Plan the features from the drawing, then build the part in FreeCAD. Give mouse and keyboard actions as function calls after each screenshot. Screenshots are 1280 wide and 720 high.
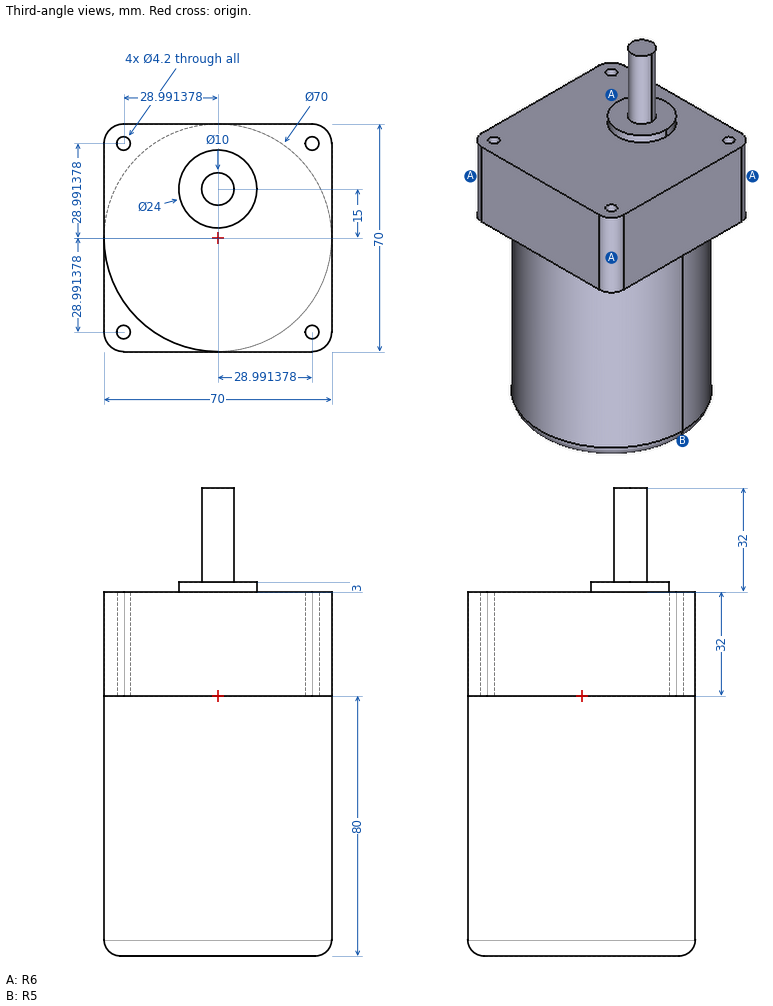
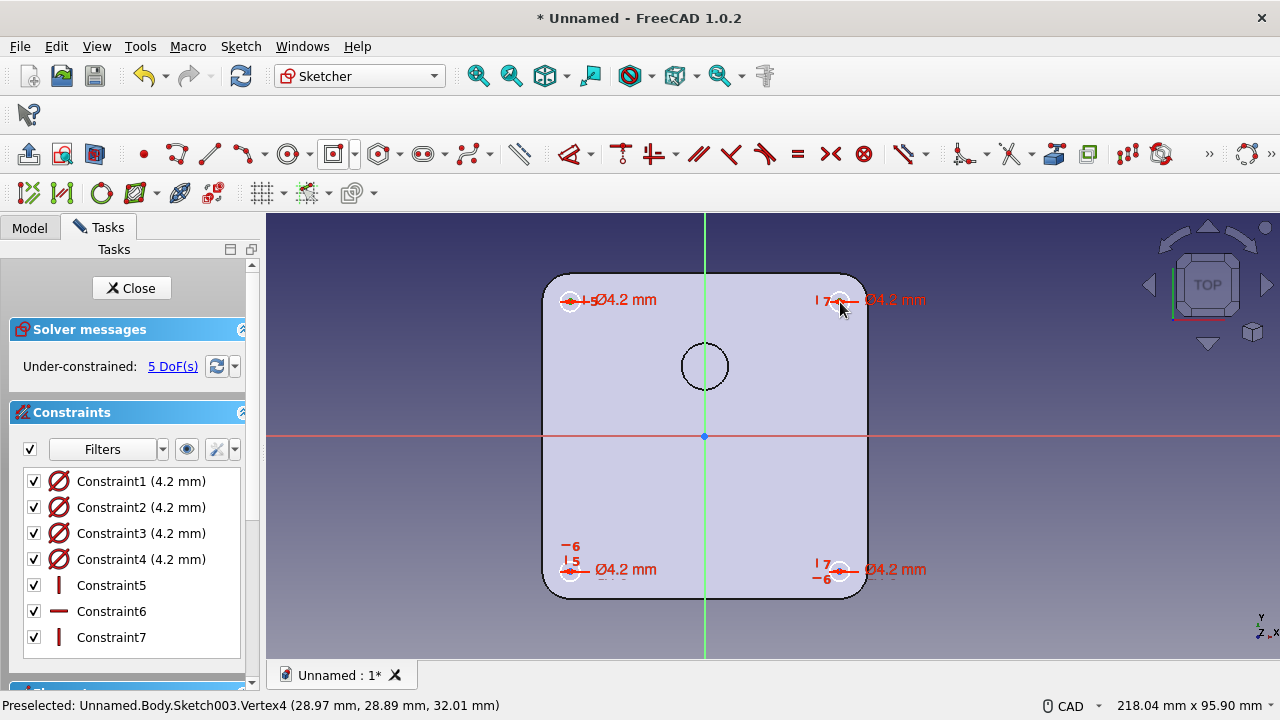
click(676, 154)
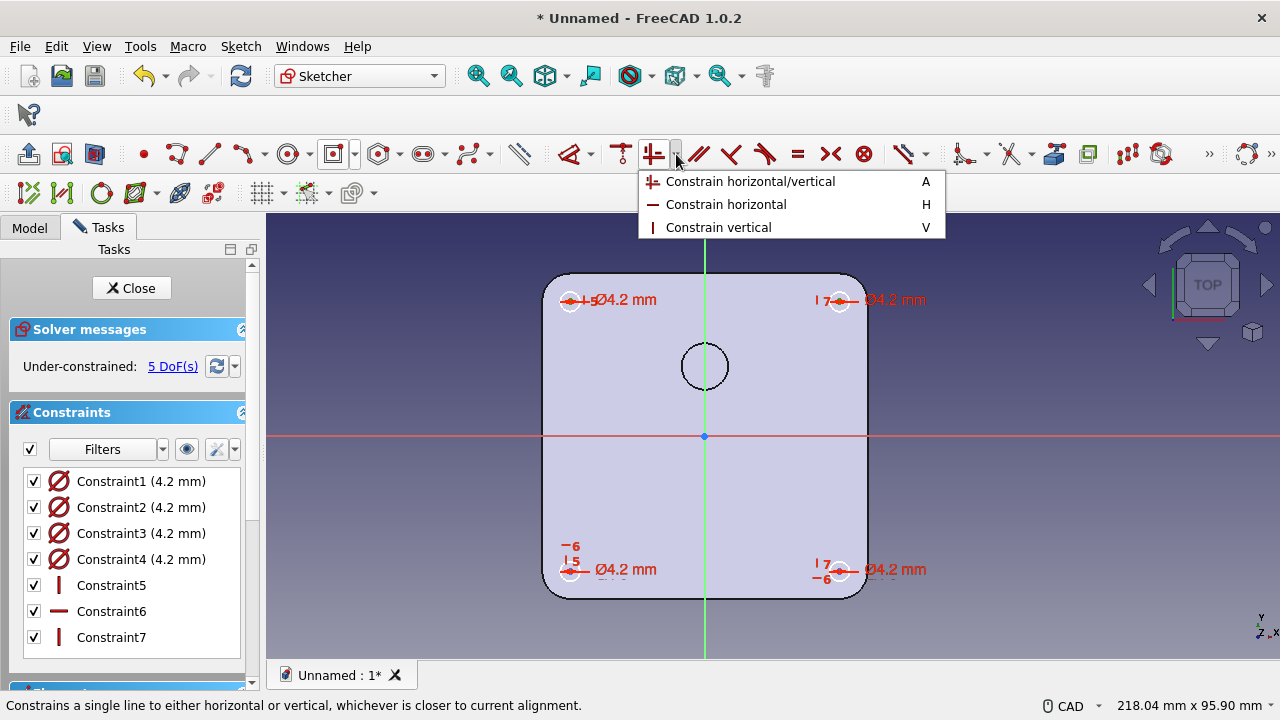
click(792, 204)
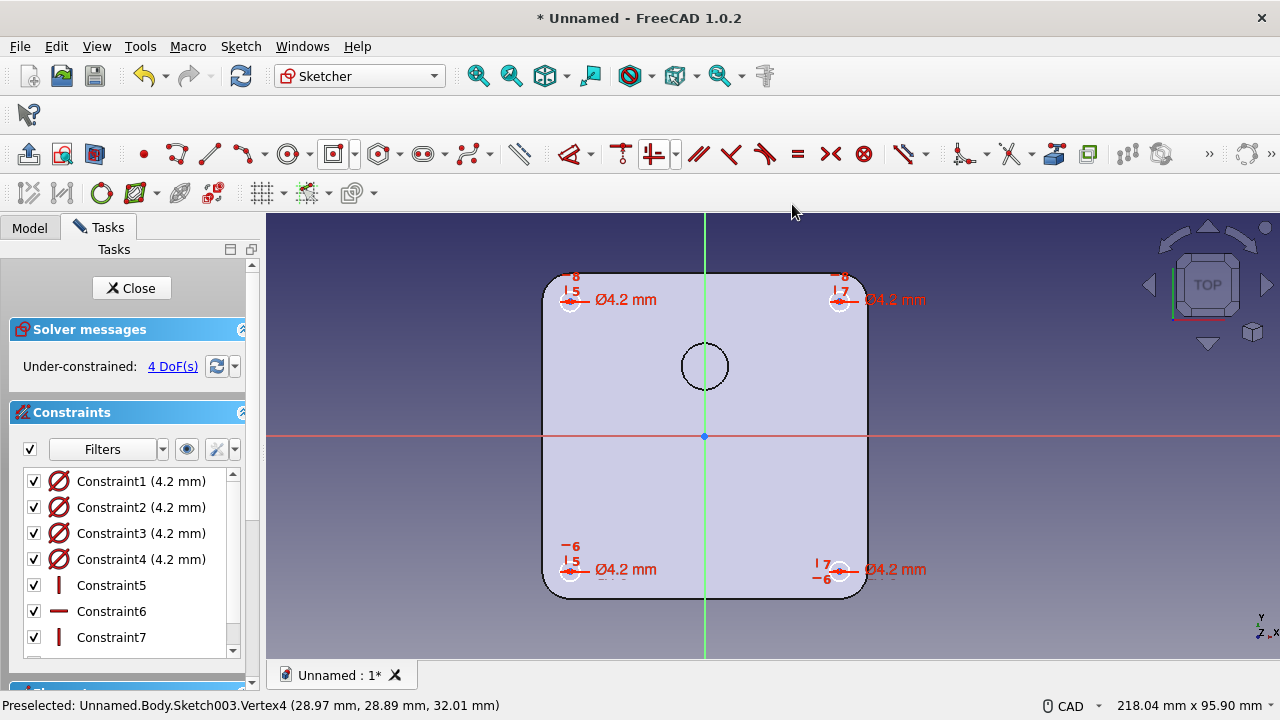
click(568, 154)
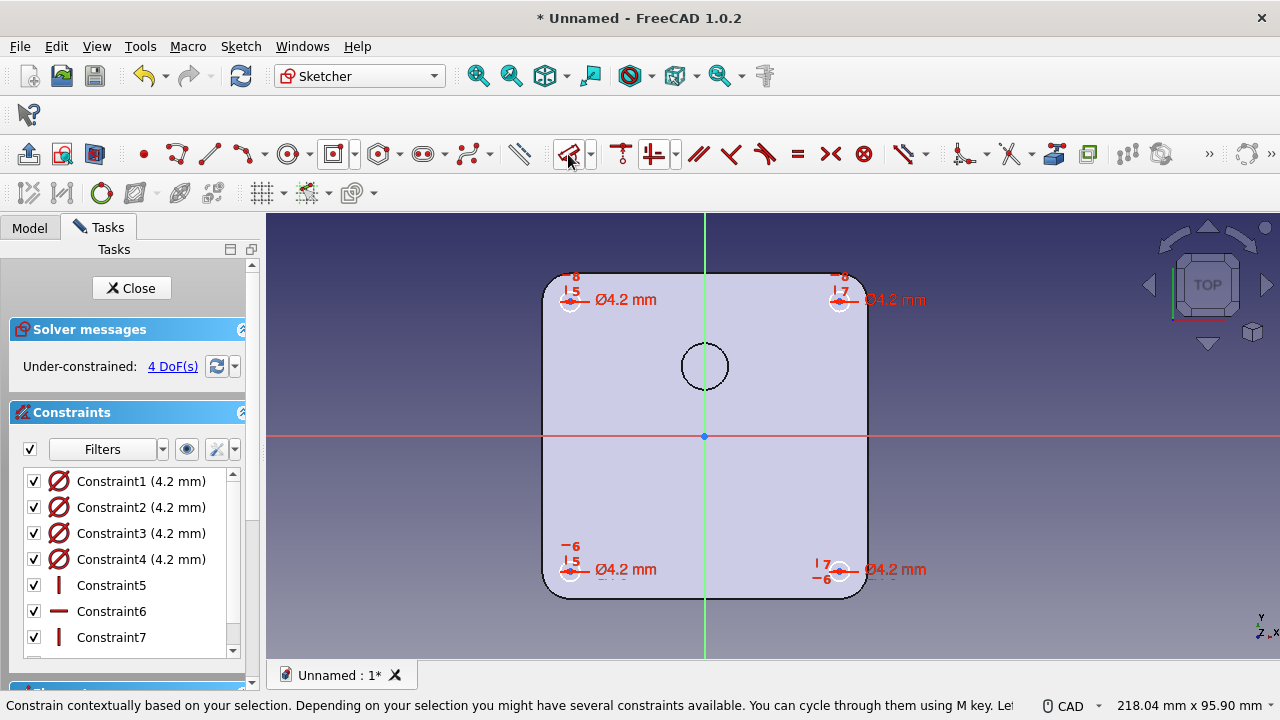
click(570, 302)
click(638, 268)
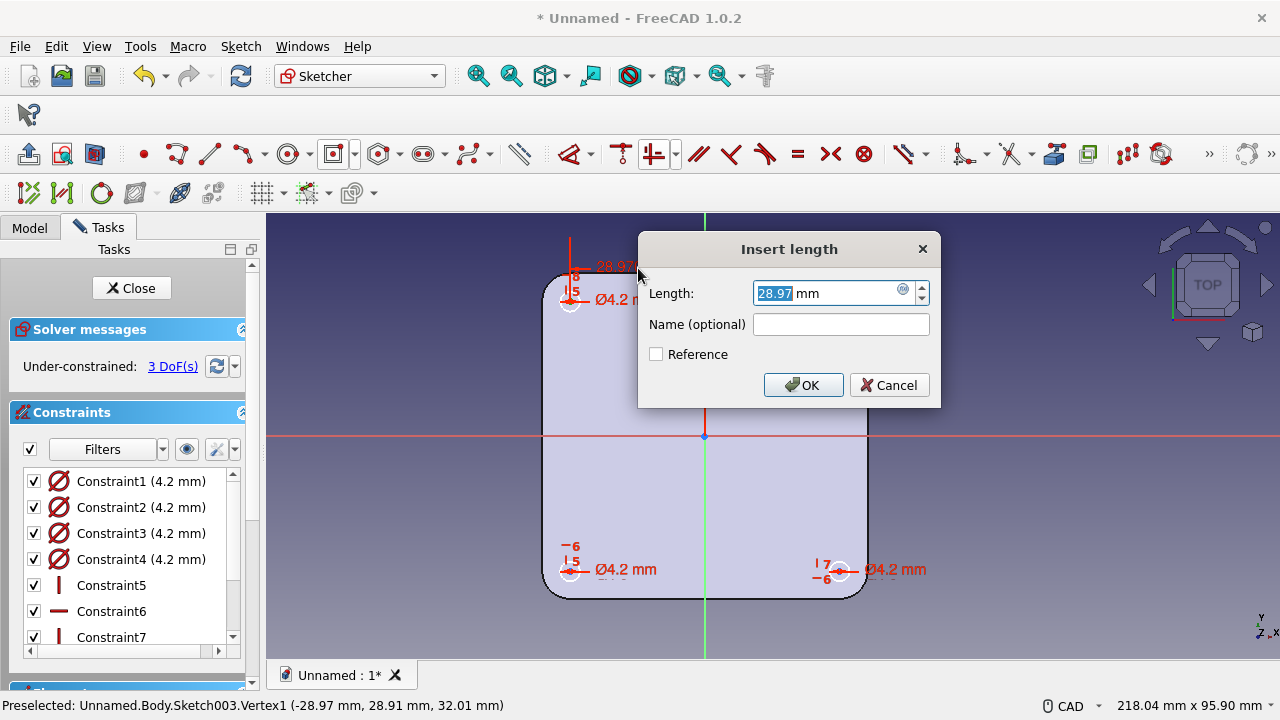
text(28.991378)
key(Return)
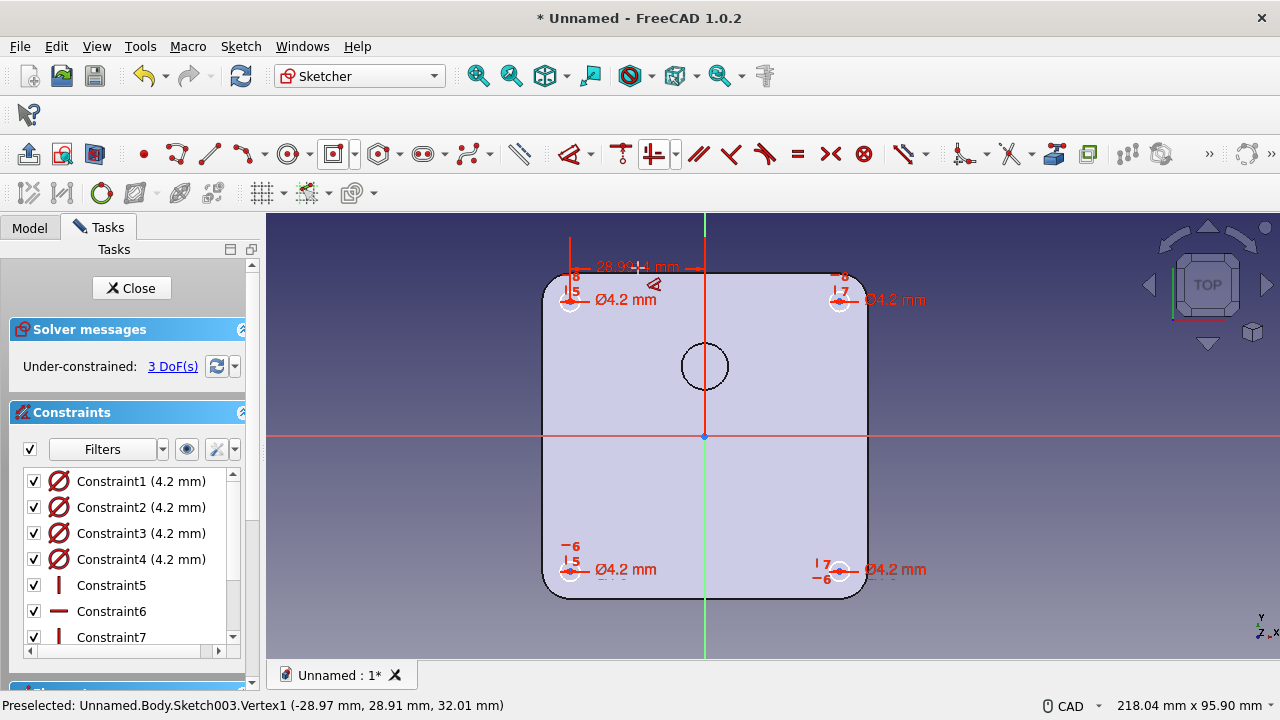
click(570, 302)
click(536, 369)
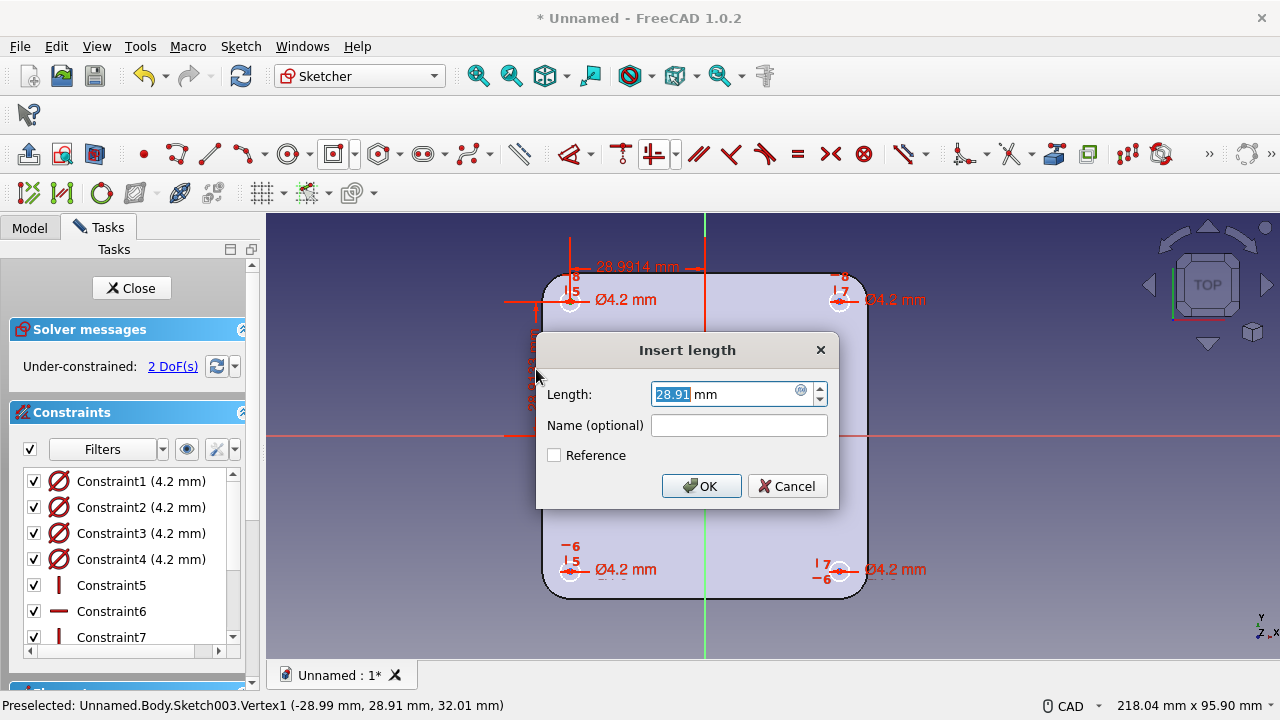
text(28.991378)
key(Return)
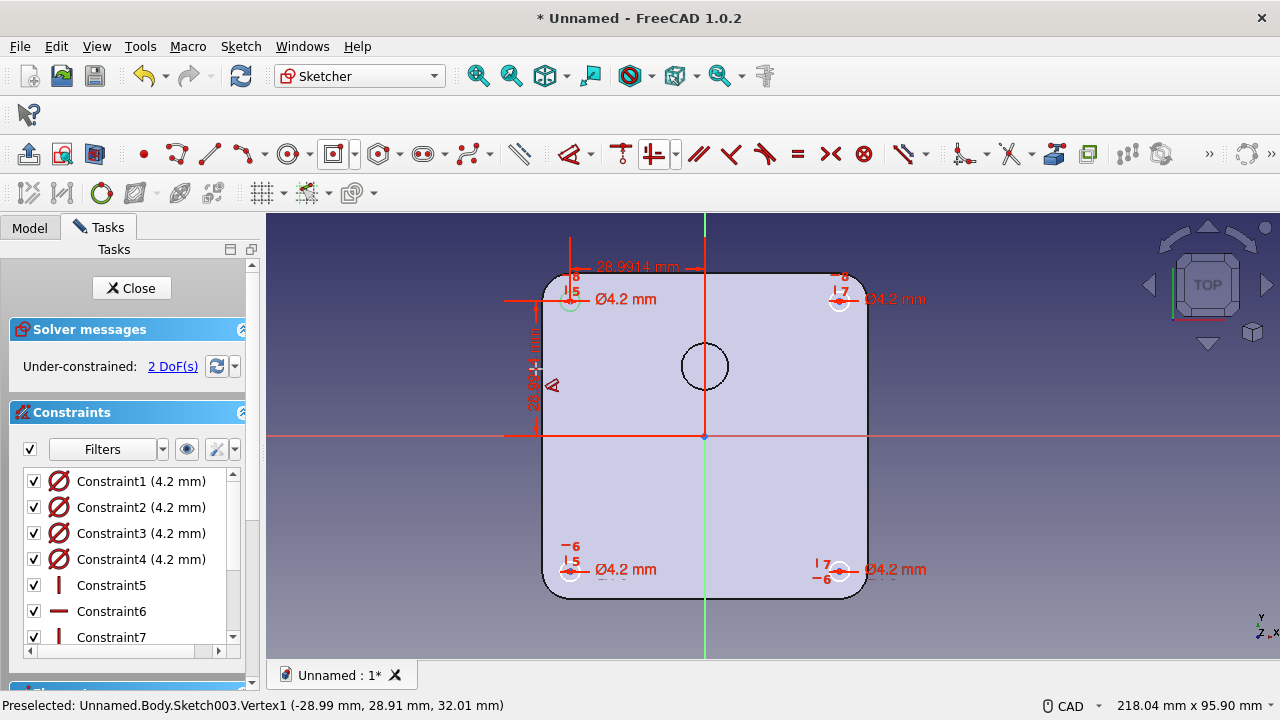
click(570, 572)
click(536, 504)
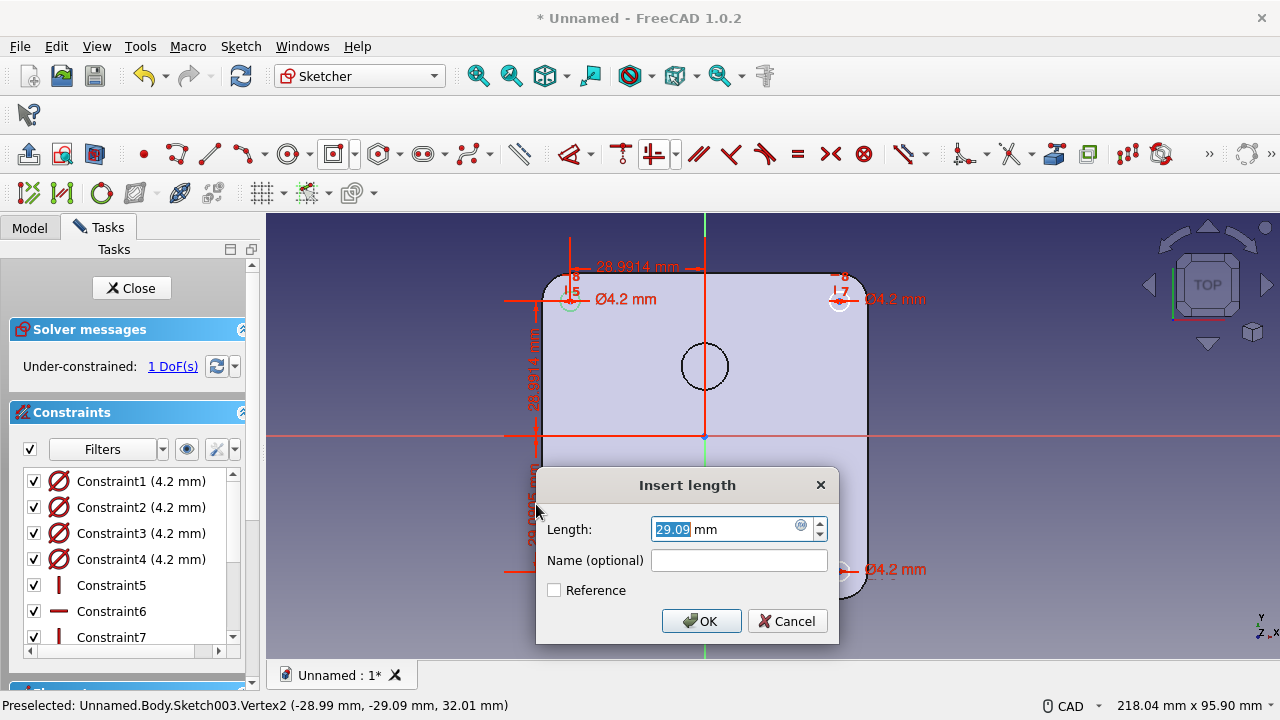
text(28.991378)
key(Return)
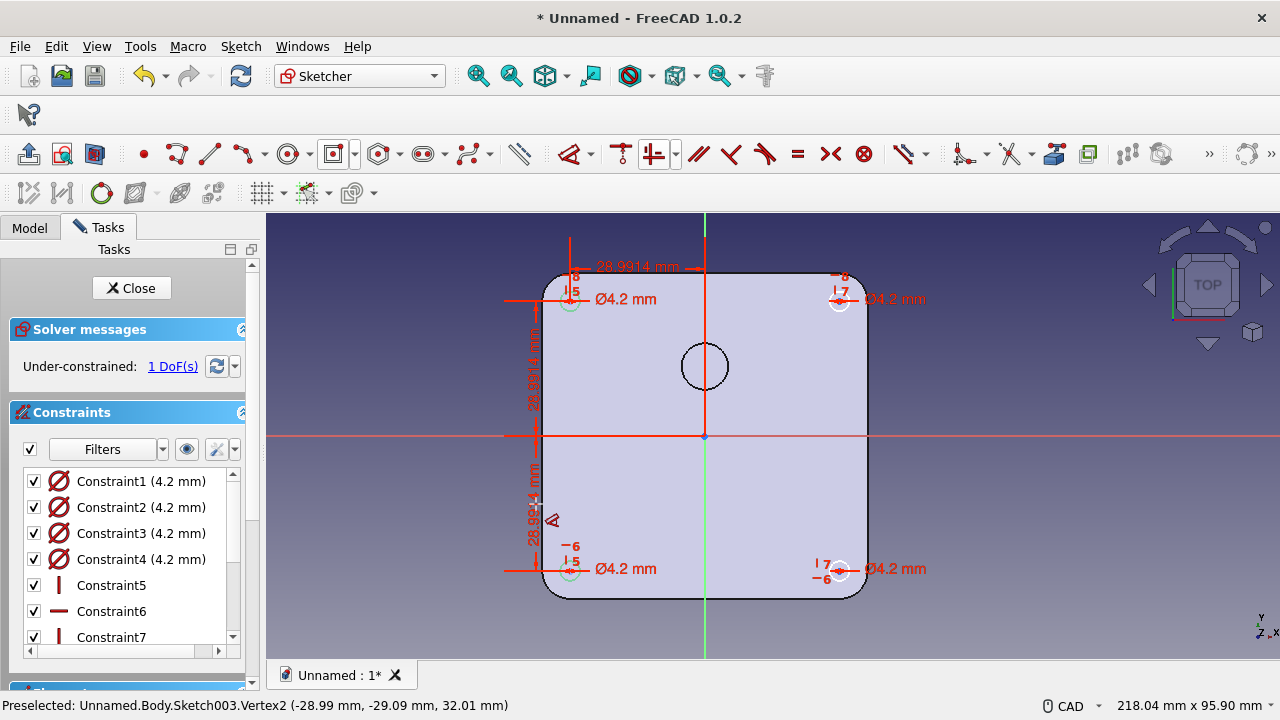
click(840, 571)
click(772, 605)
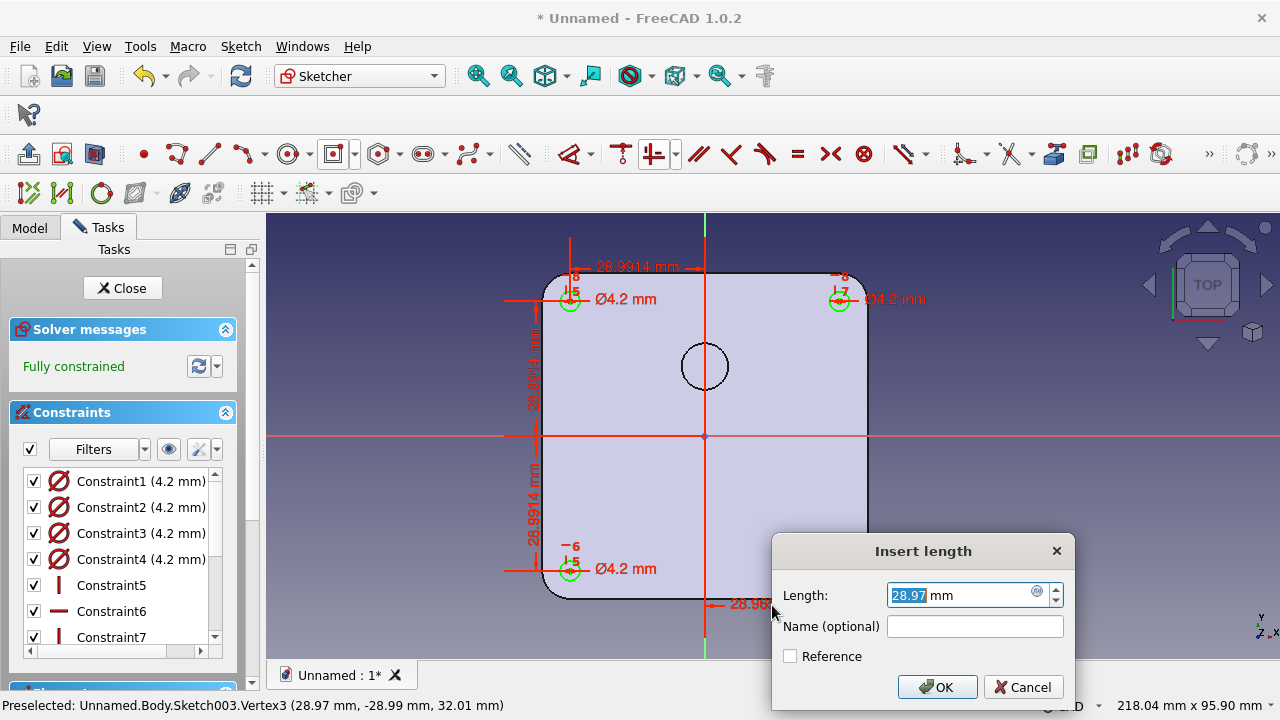
text(28.991378)
key(Return)
key(Escape)